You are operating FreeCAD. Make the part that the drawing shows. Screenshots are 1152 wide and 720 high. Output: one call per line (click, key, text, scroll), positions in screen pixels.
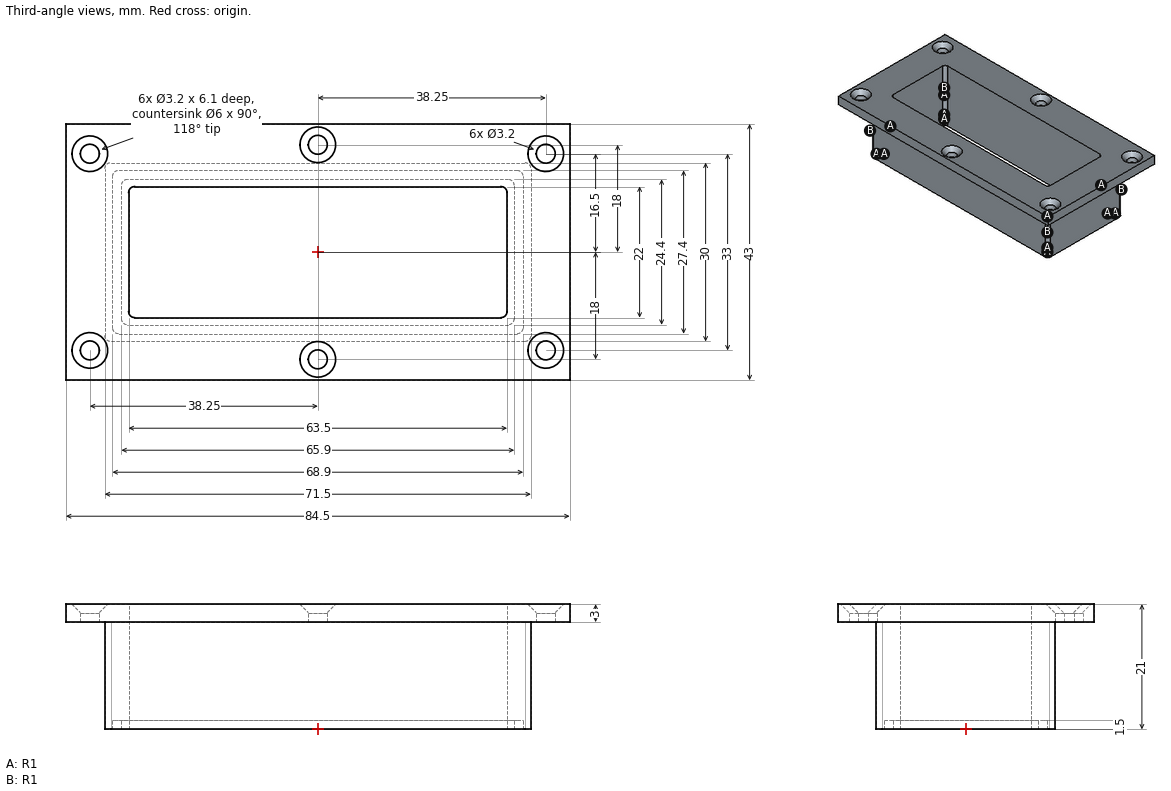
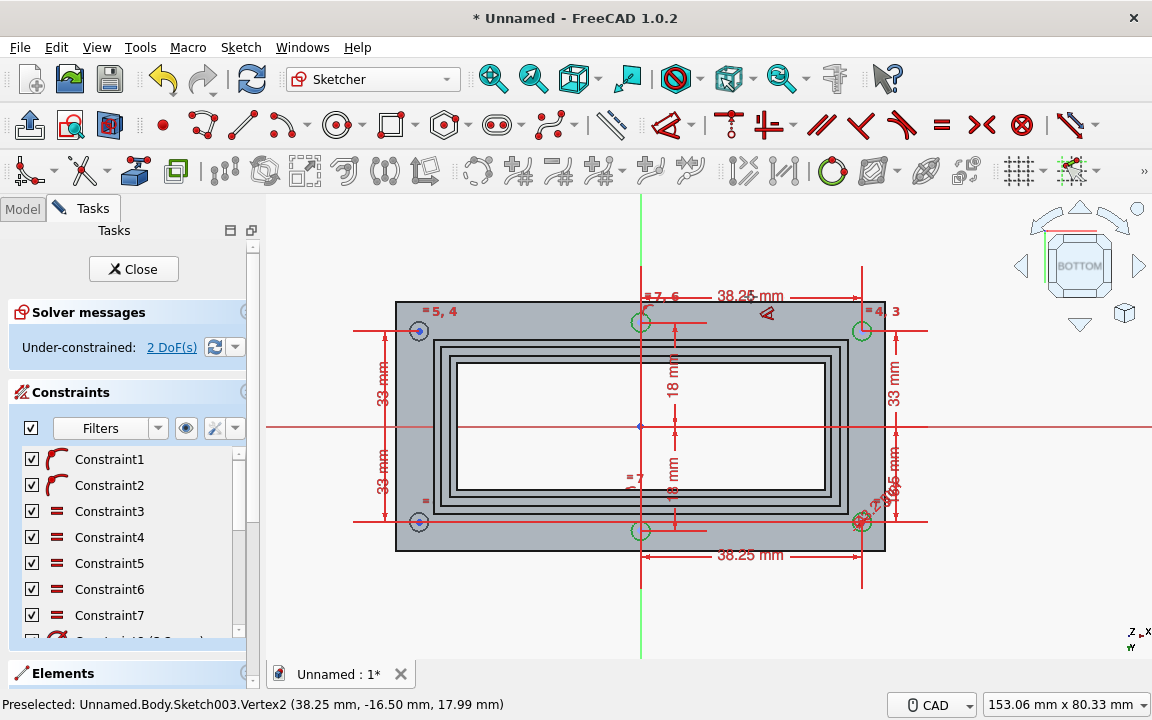
click(419, 331)
click(530, 297)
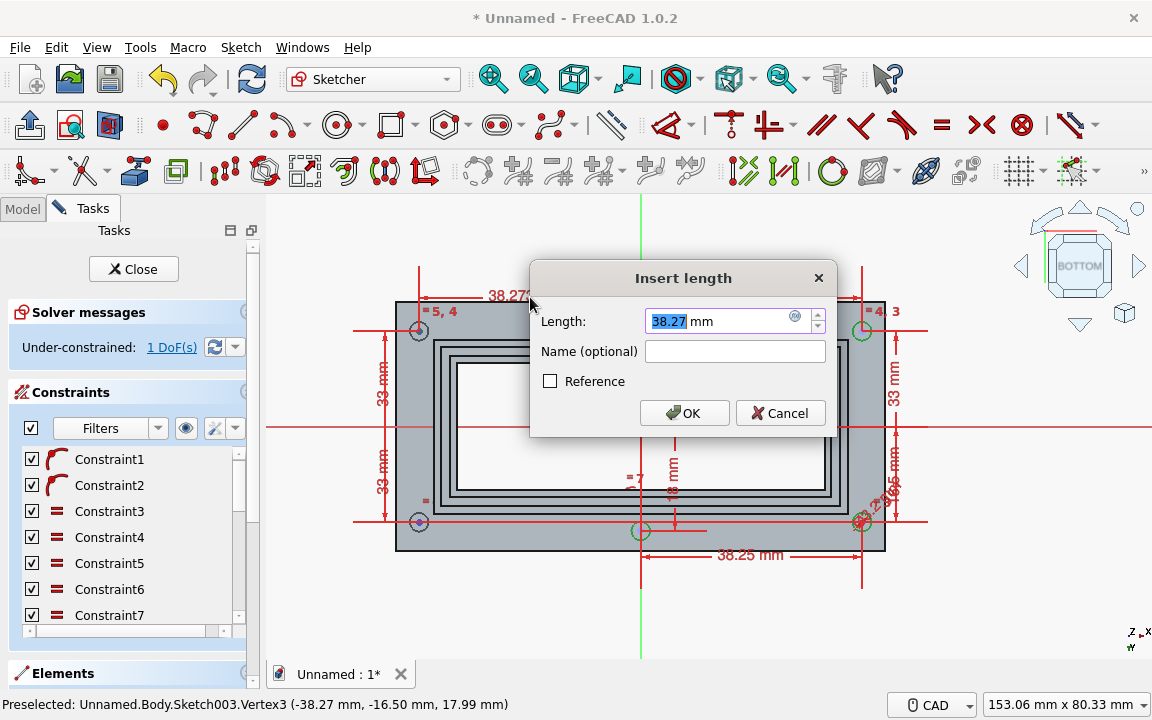
text(38.25)
key(Return)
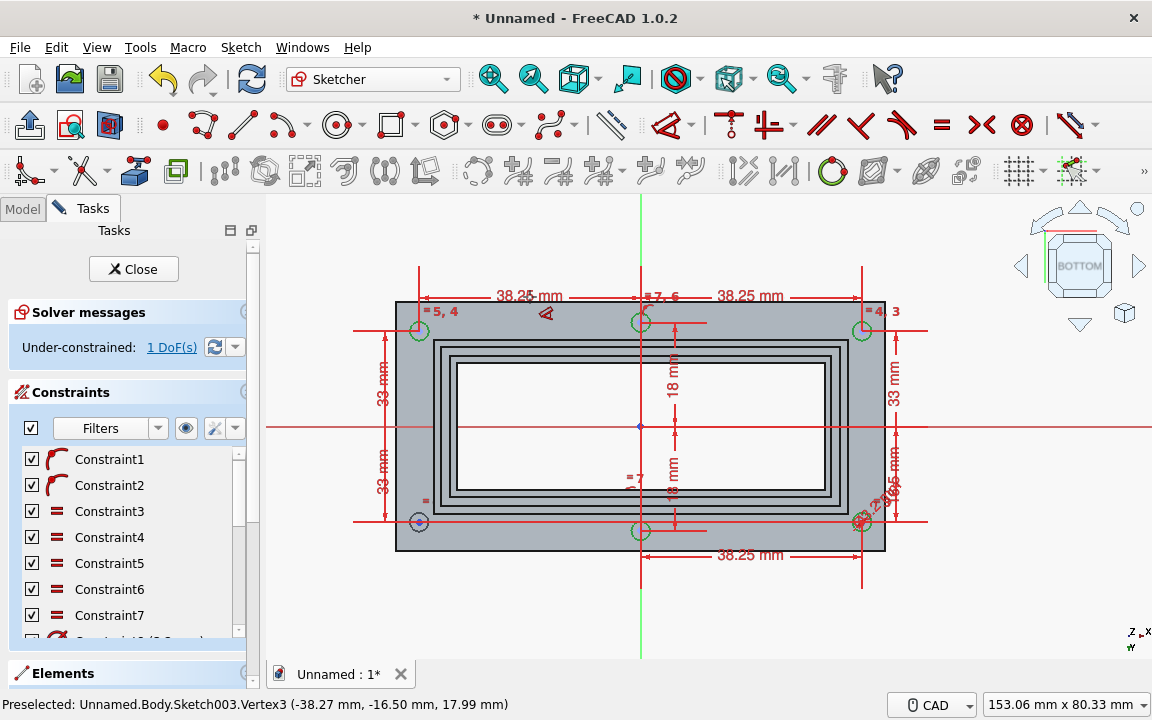
click(419, 522)
click(530, 556)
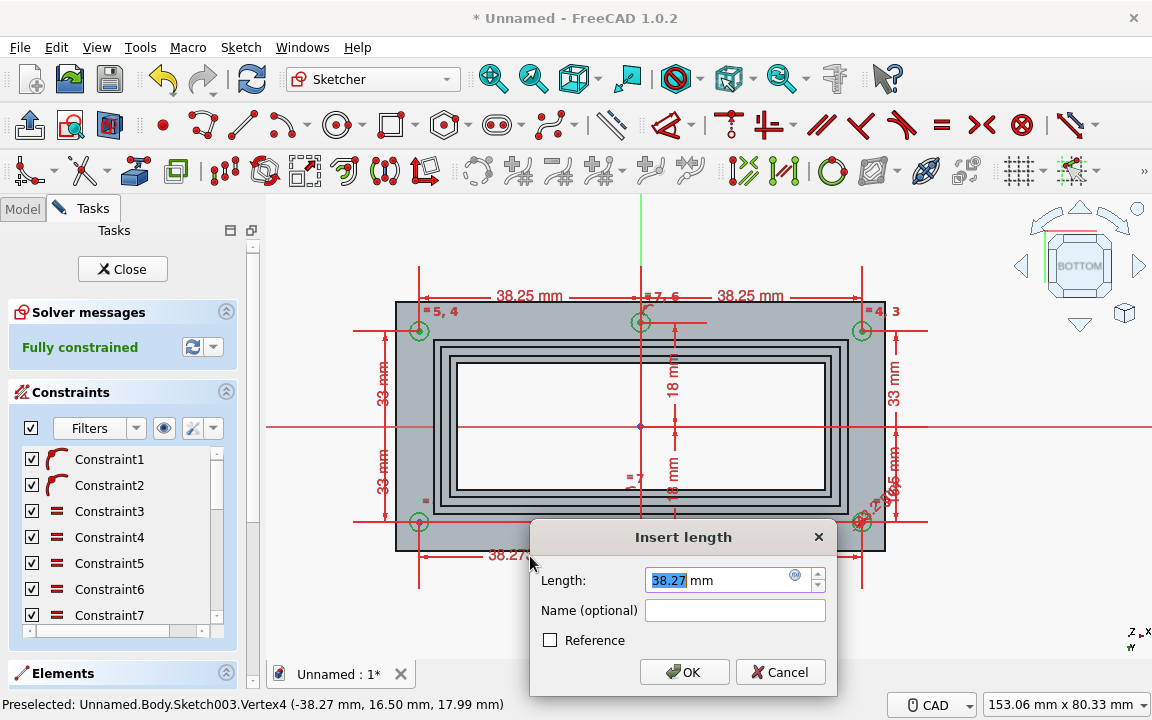
text(38.25)
key(Return)
key(Escape)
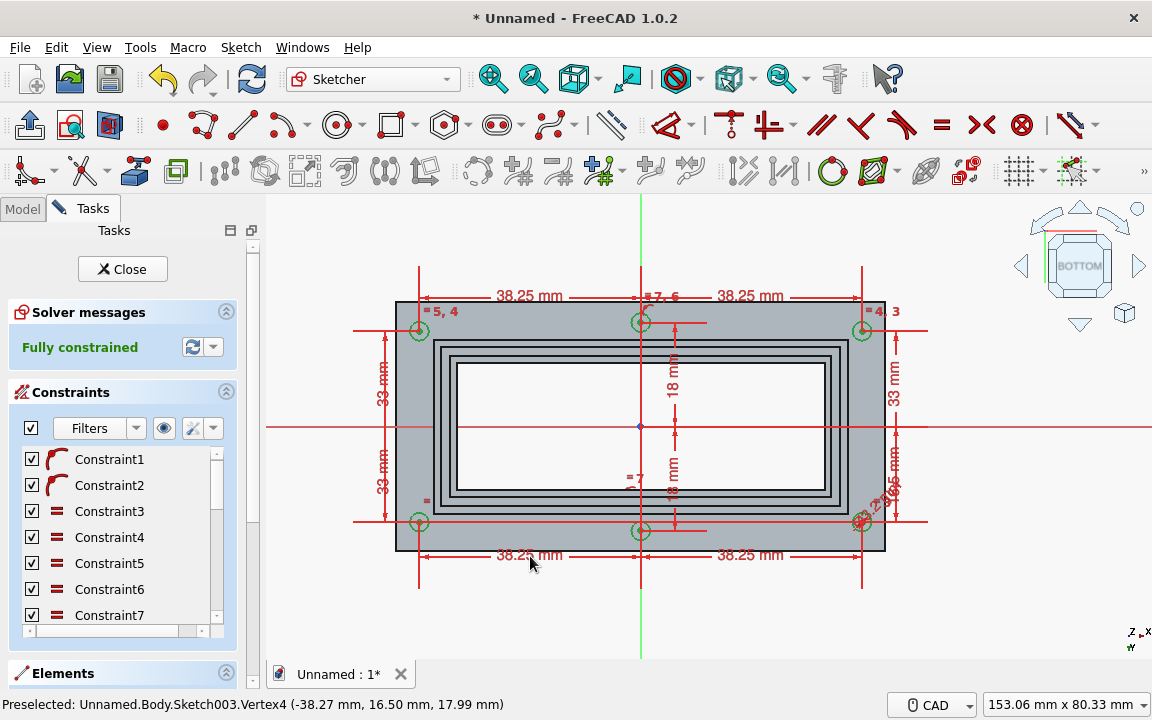
click(123, 269)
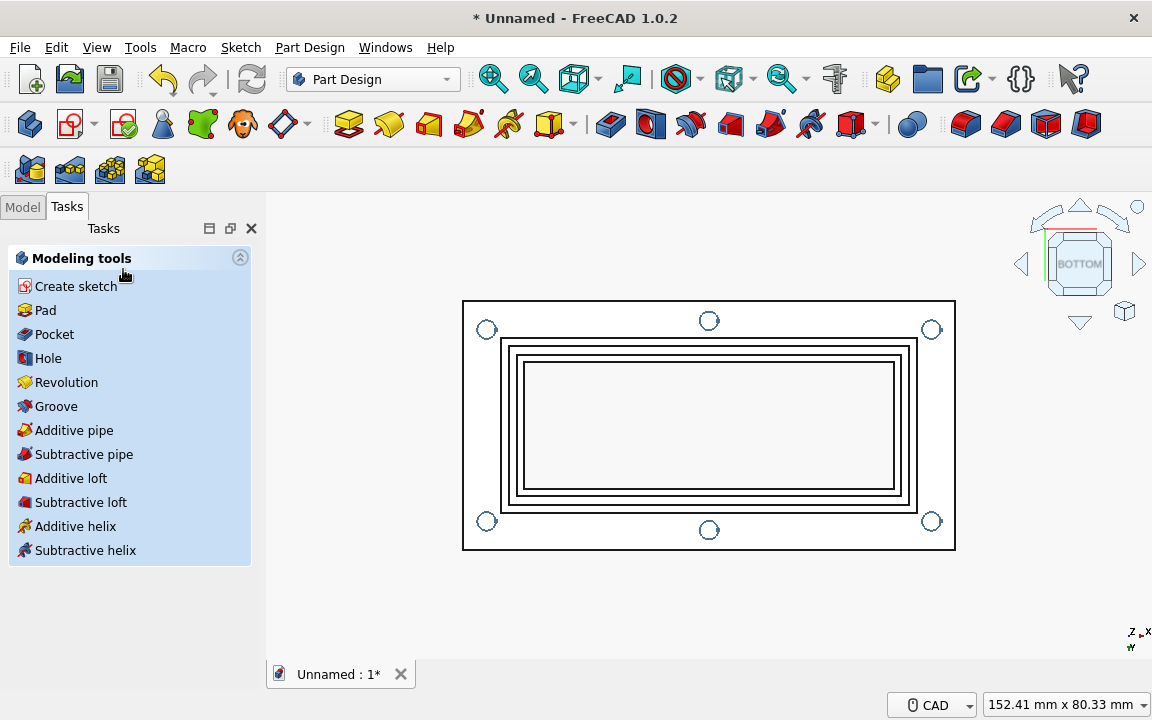
click(612, 124)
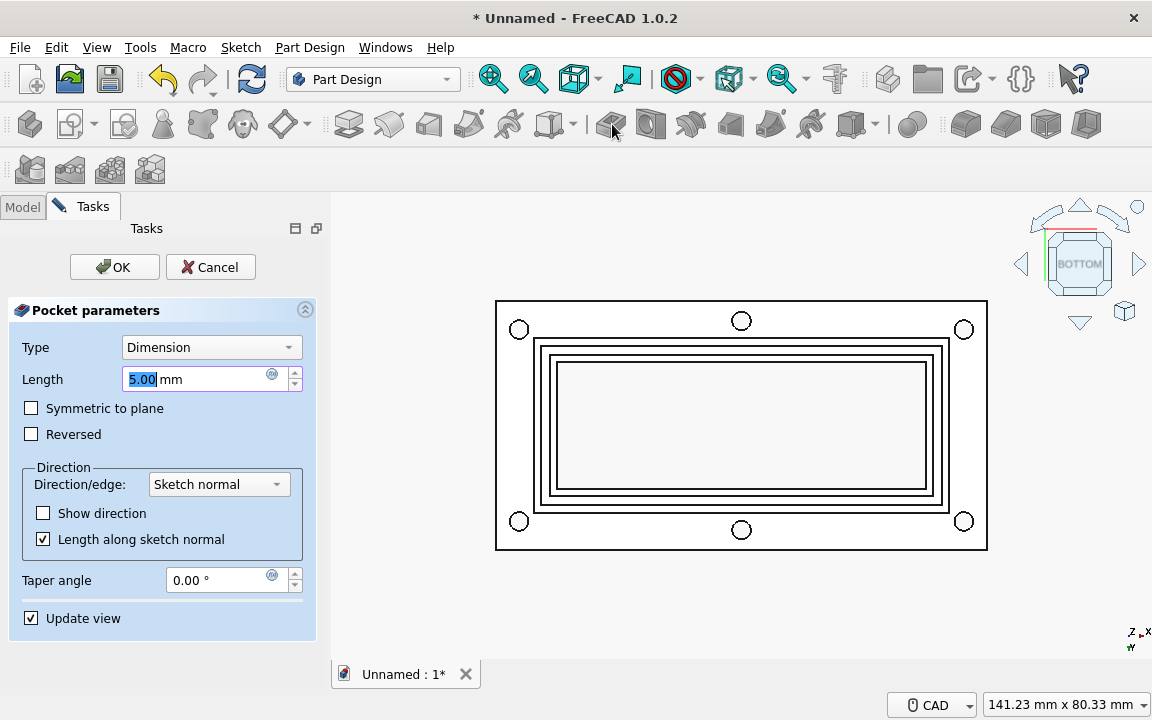
text(3)
key(Tab)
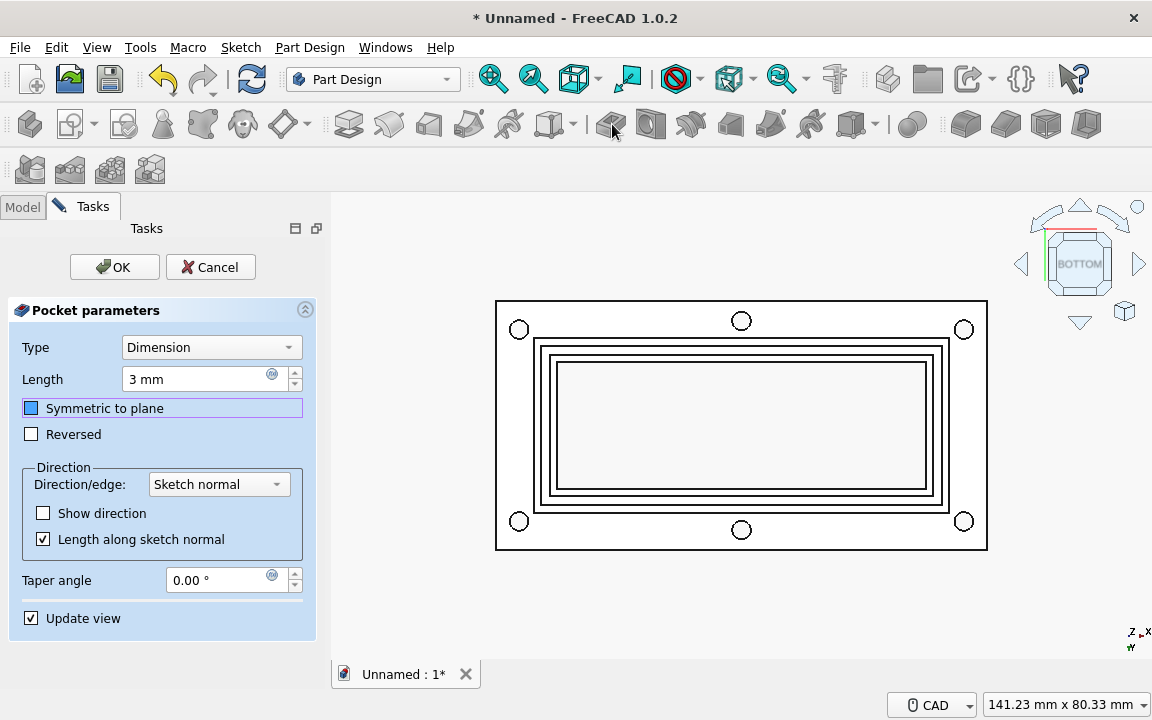
click(115, 267)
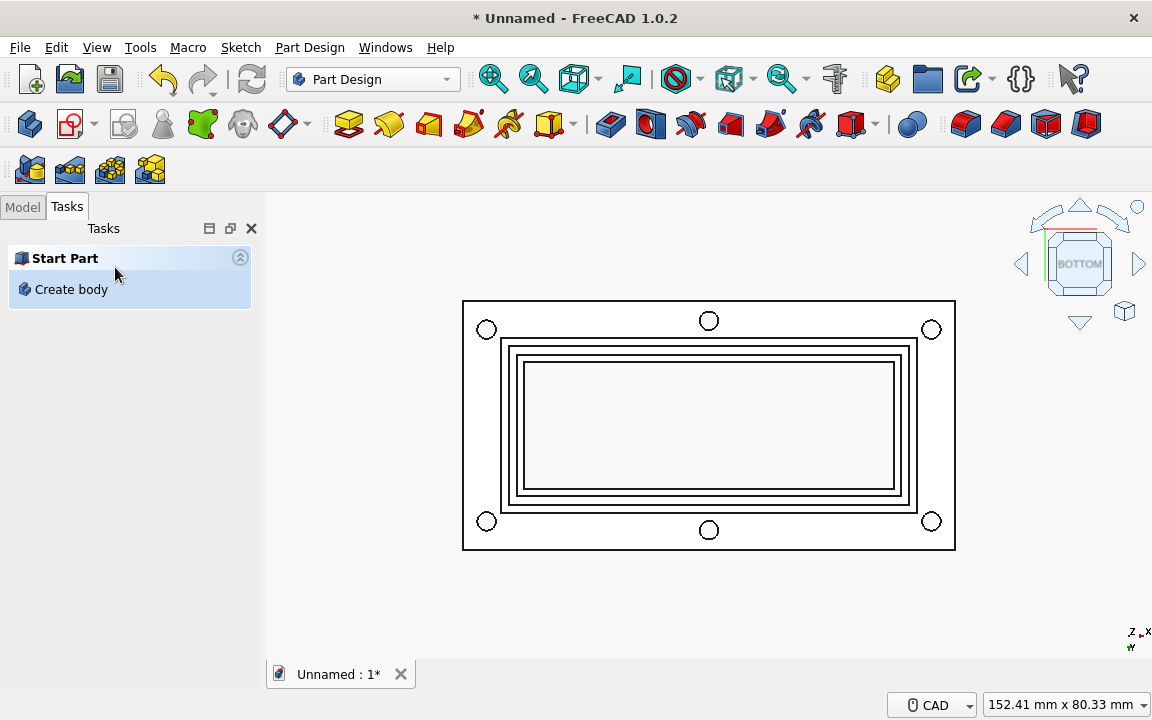
key(0)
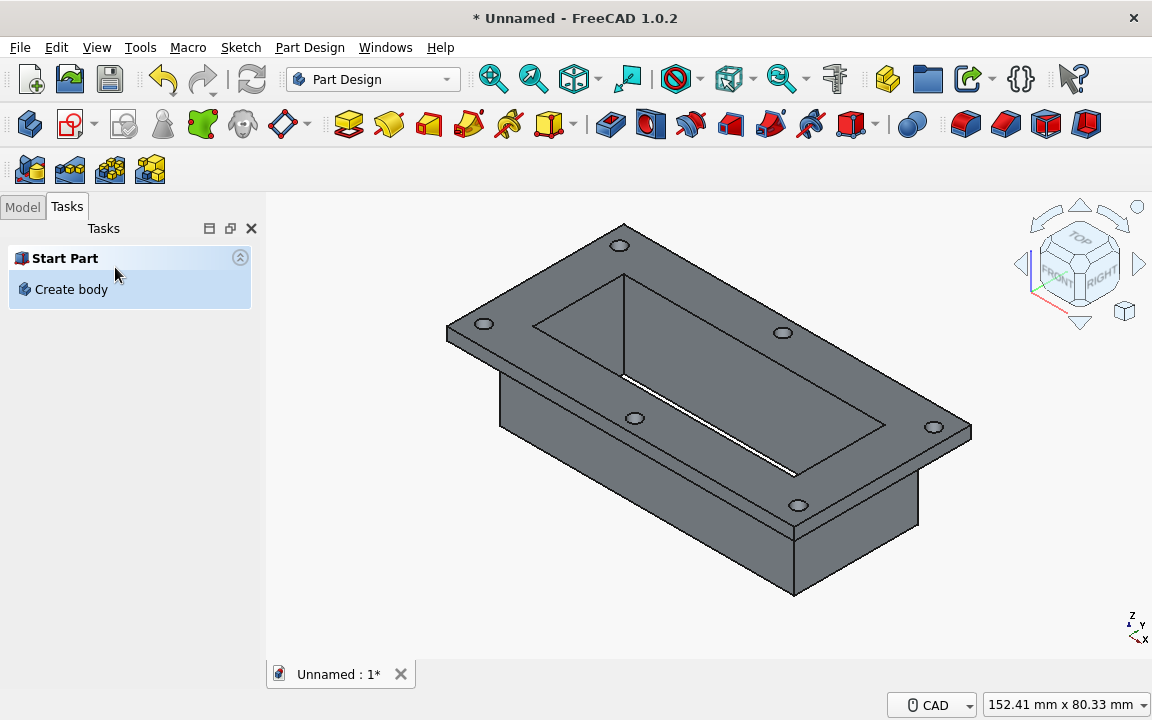
click(585, 274)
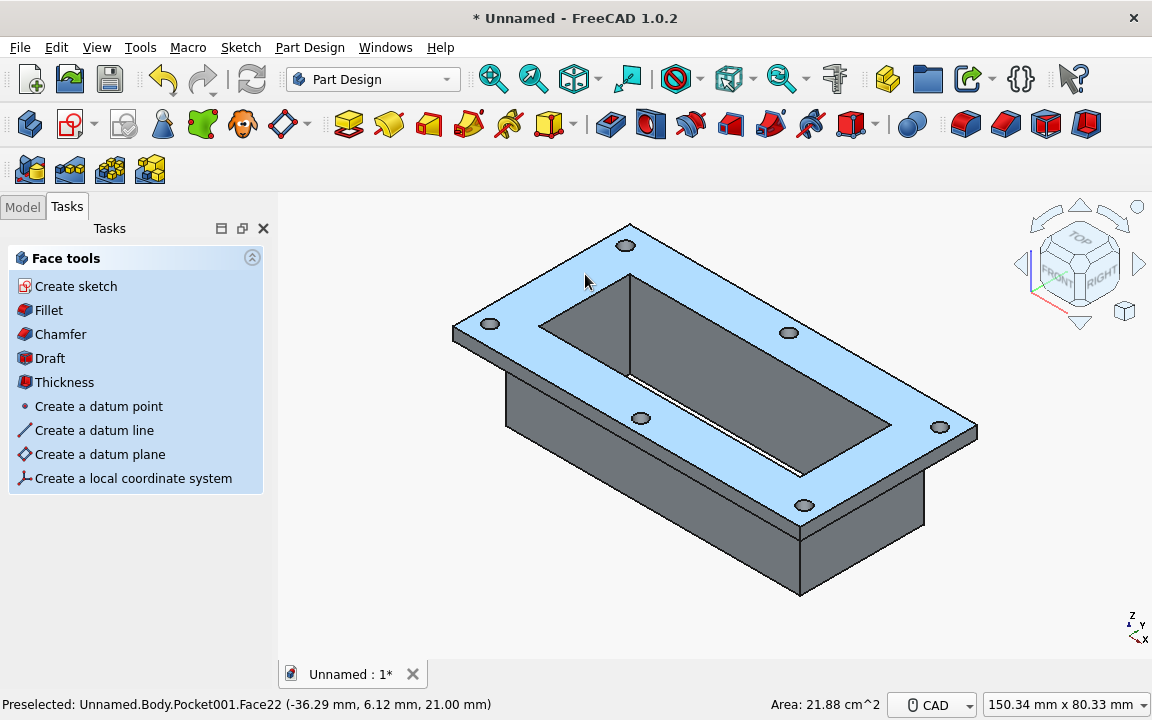
click(70, 124)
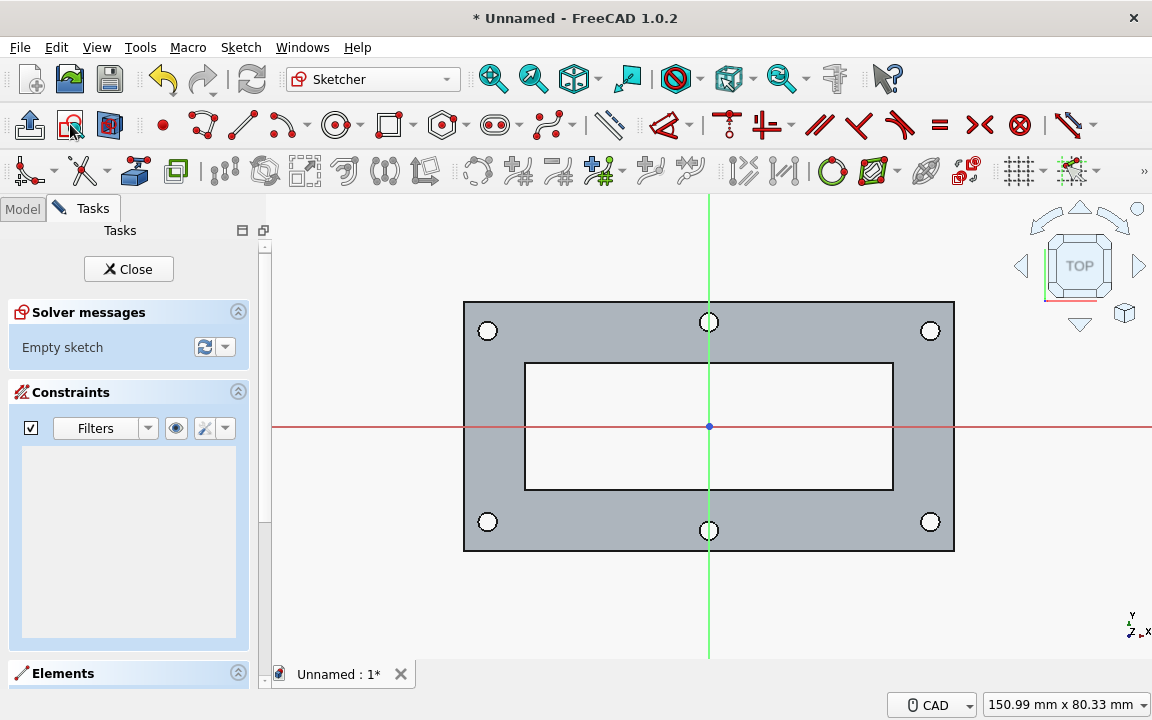
click(336, 126)